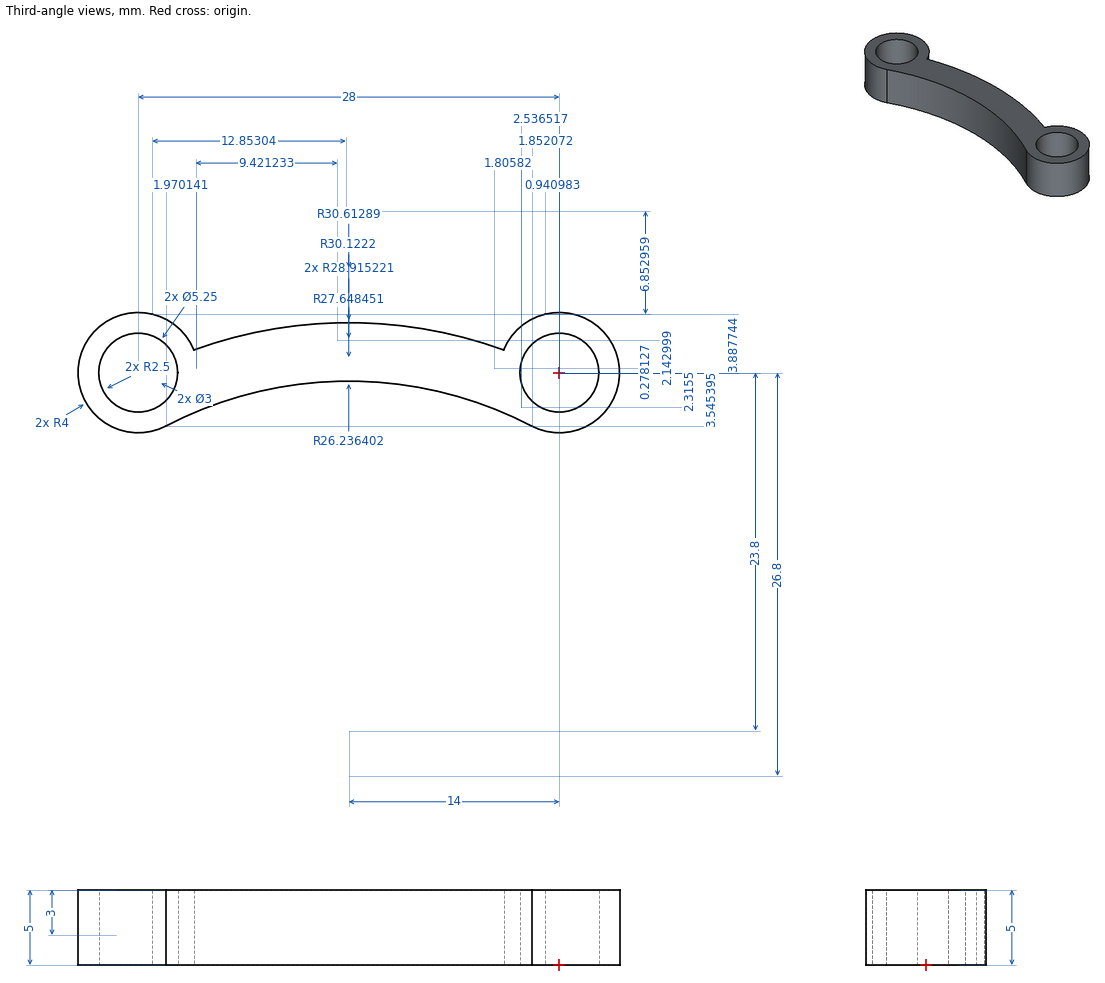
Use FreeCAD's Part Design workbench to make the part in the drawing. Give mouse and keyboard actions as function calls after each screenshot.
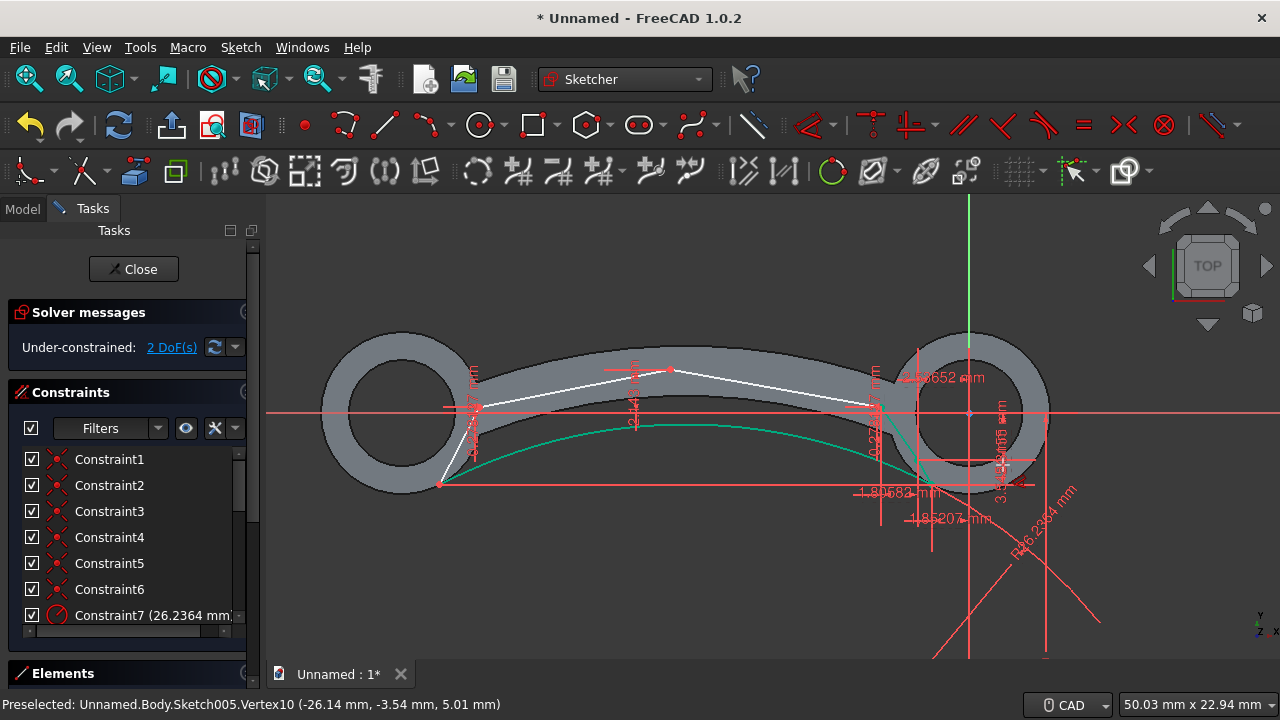
click(613, 381)
click(575, 336)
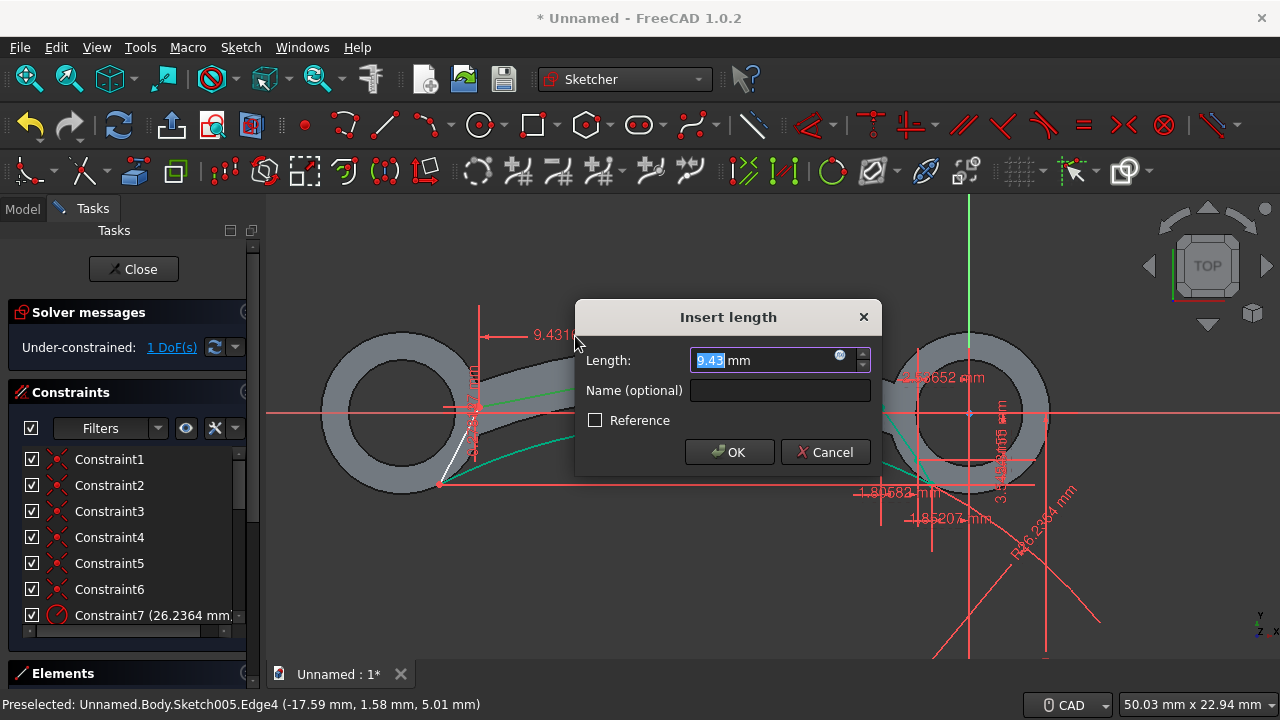
text(9.421233)
key(Return)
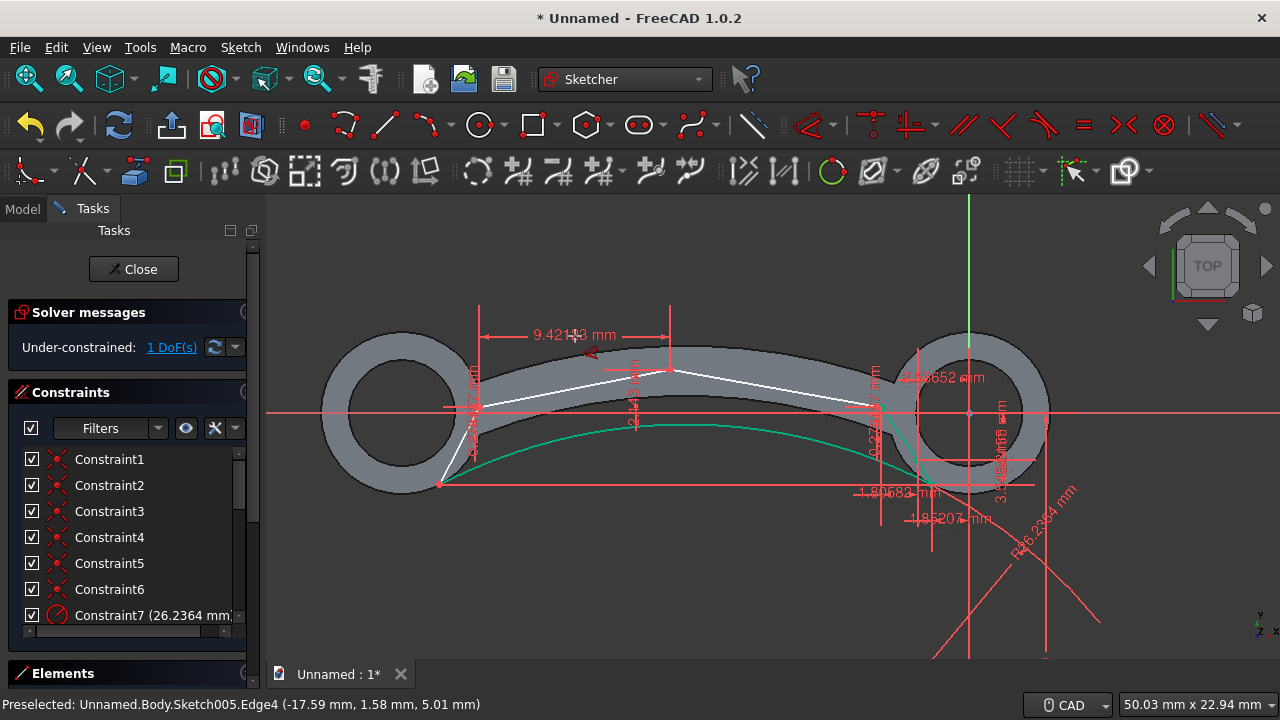
click(467, 431)
click(459, 519)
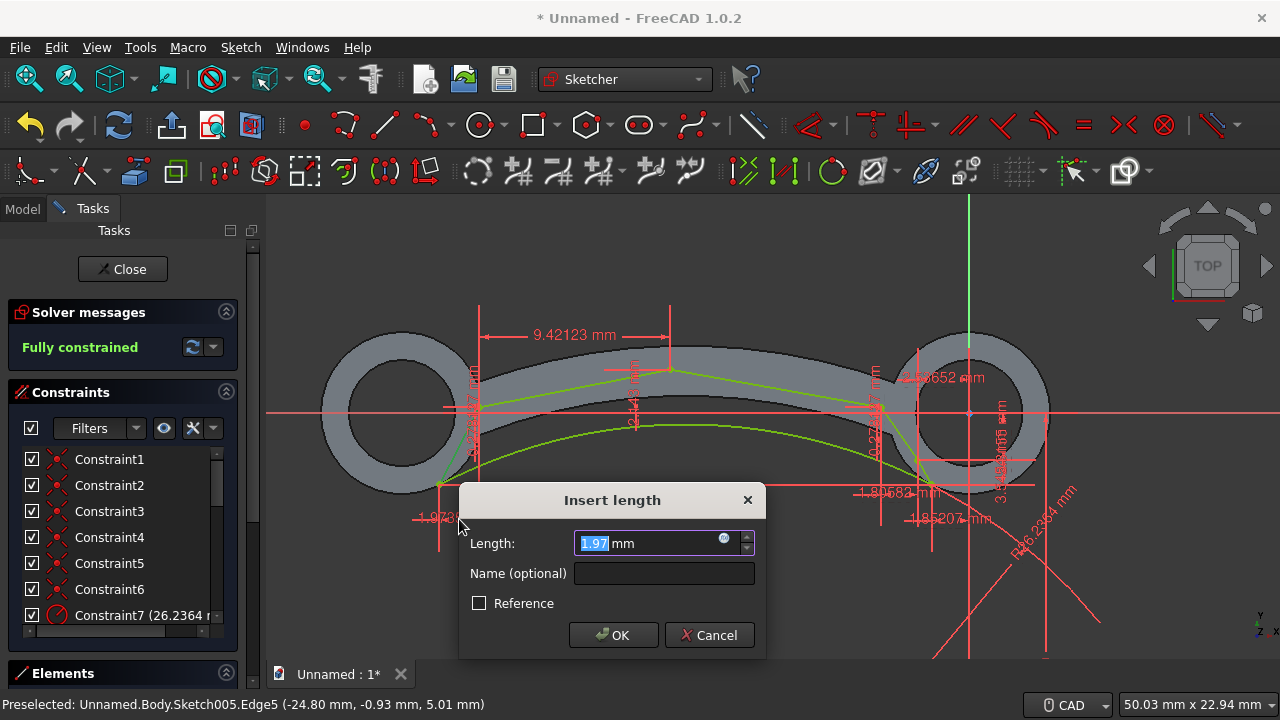
text(1.970141)
key(Return)
key(Escape)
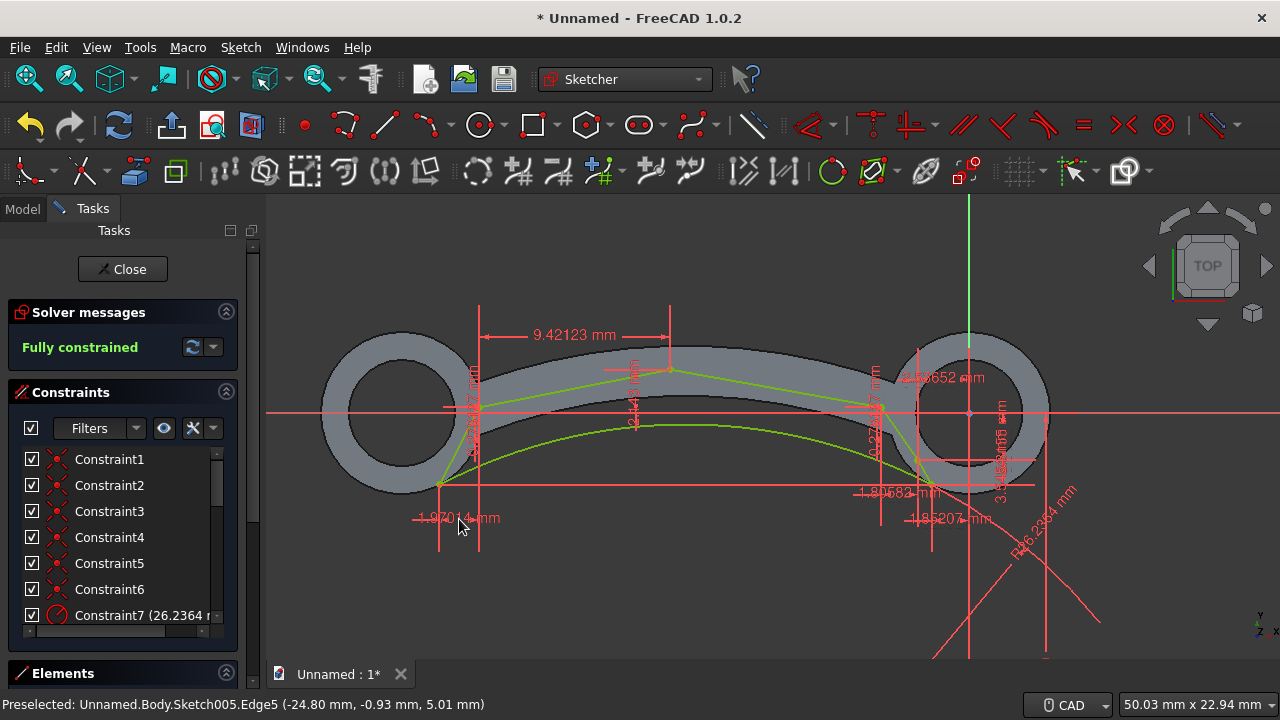
click(123, 269)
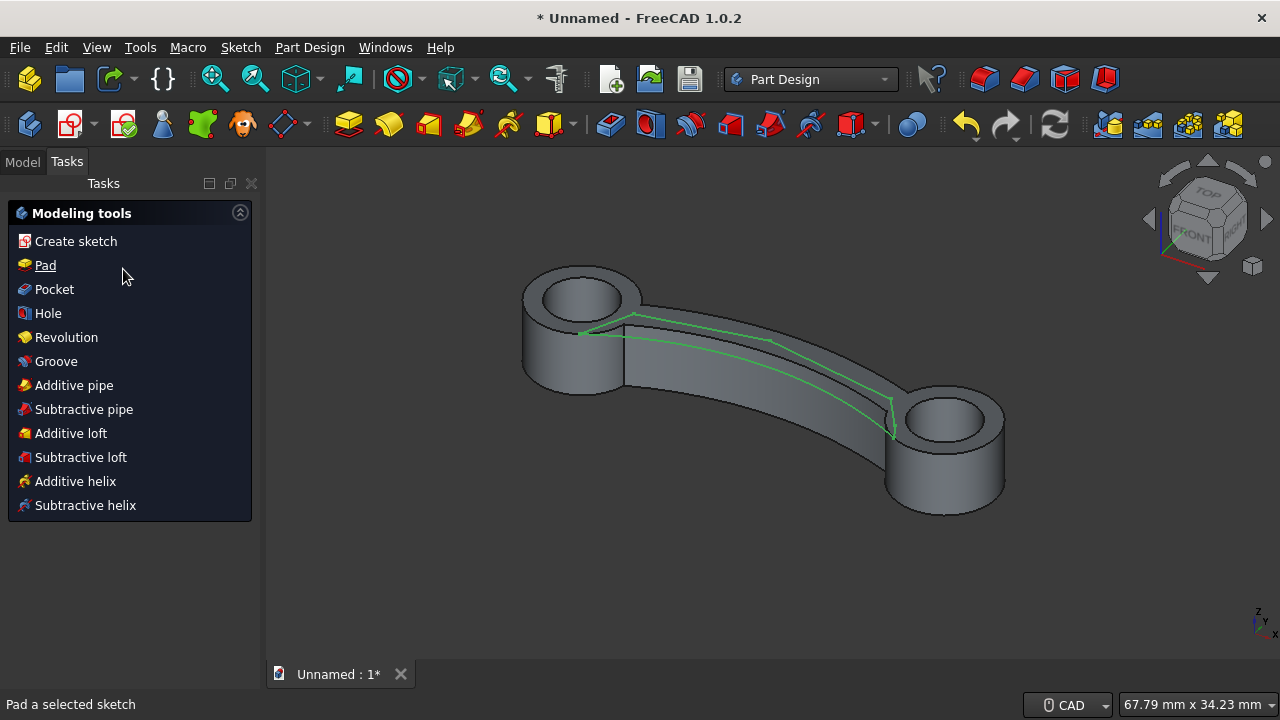
click(350, 124)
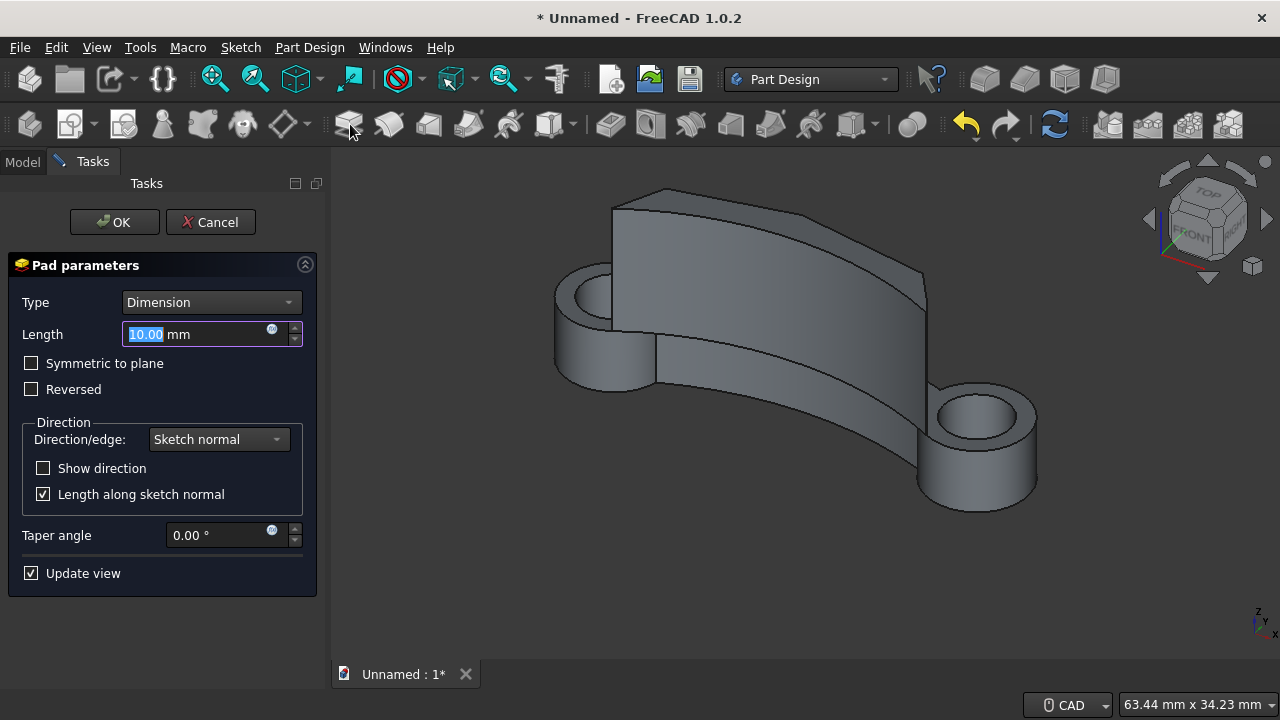
text(5)
key(Tab)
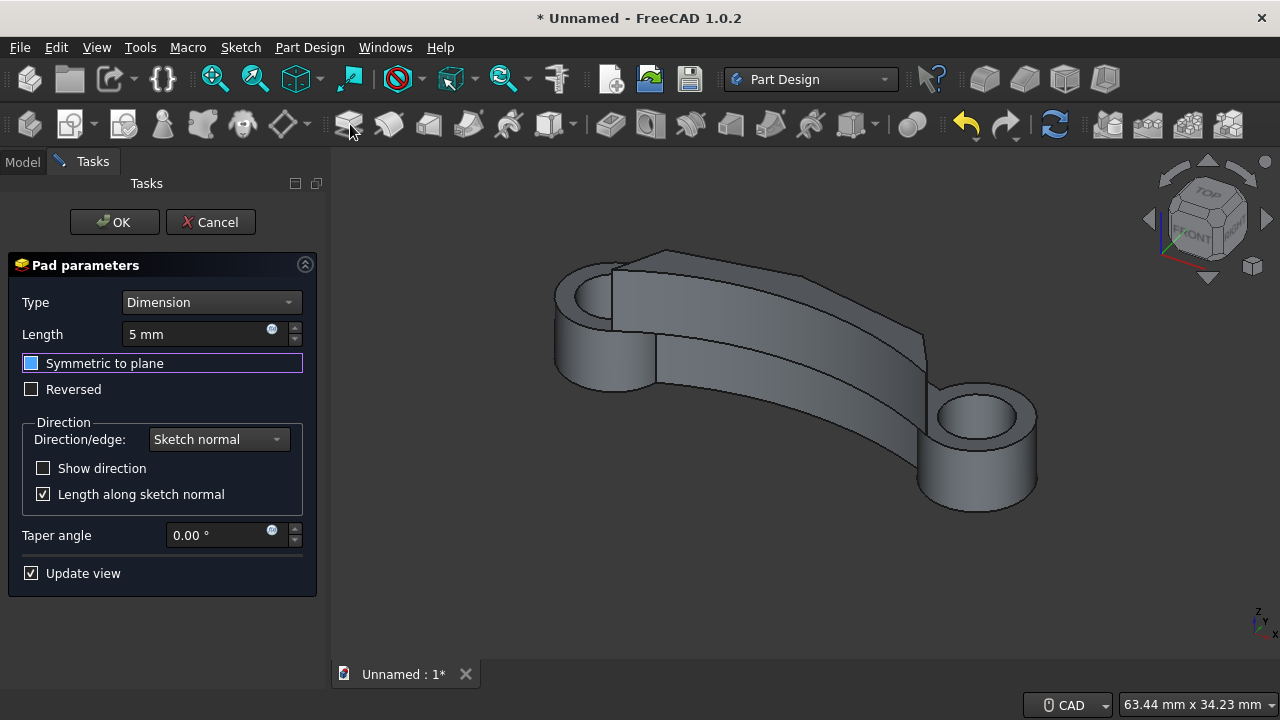
click(30, 389)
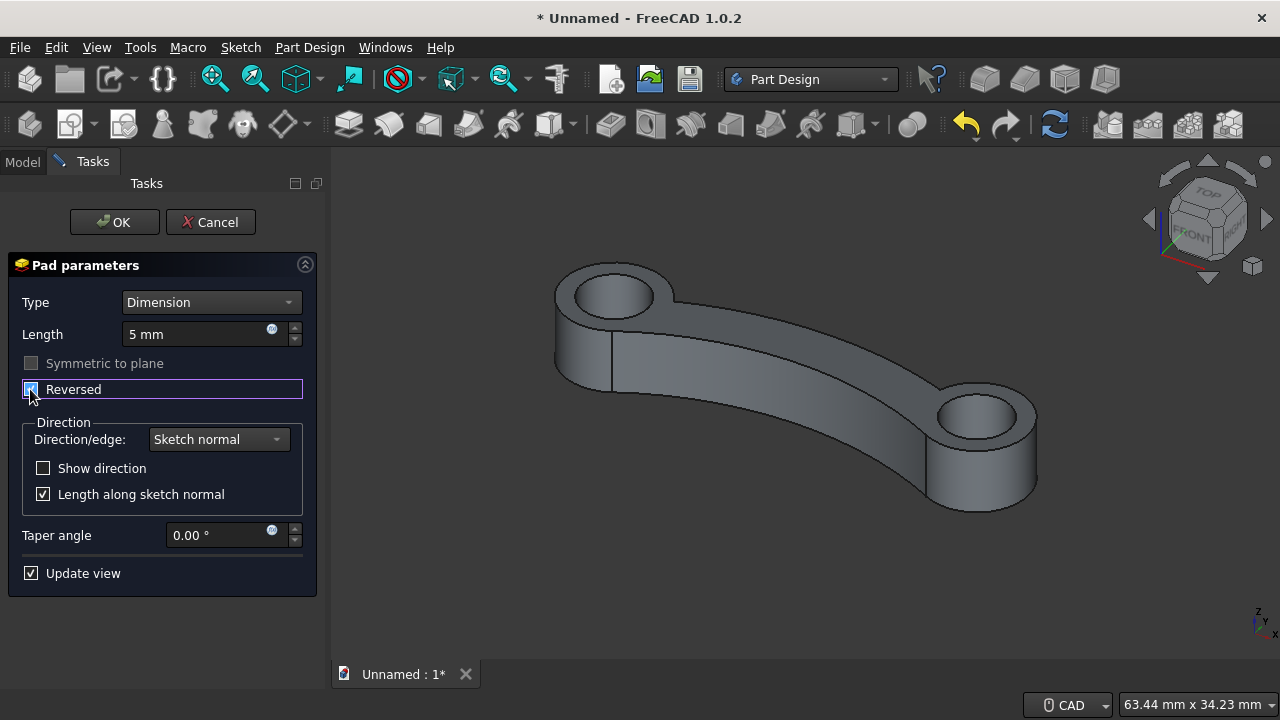
click(115, 222)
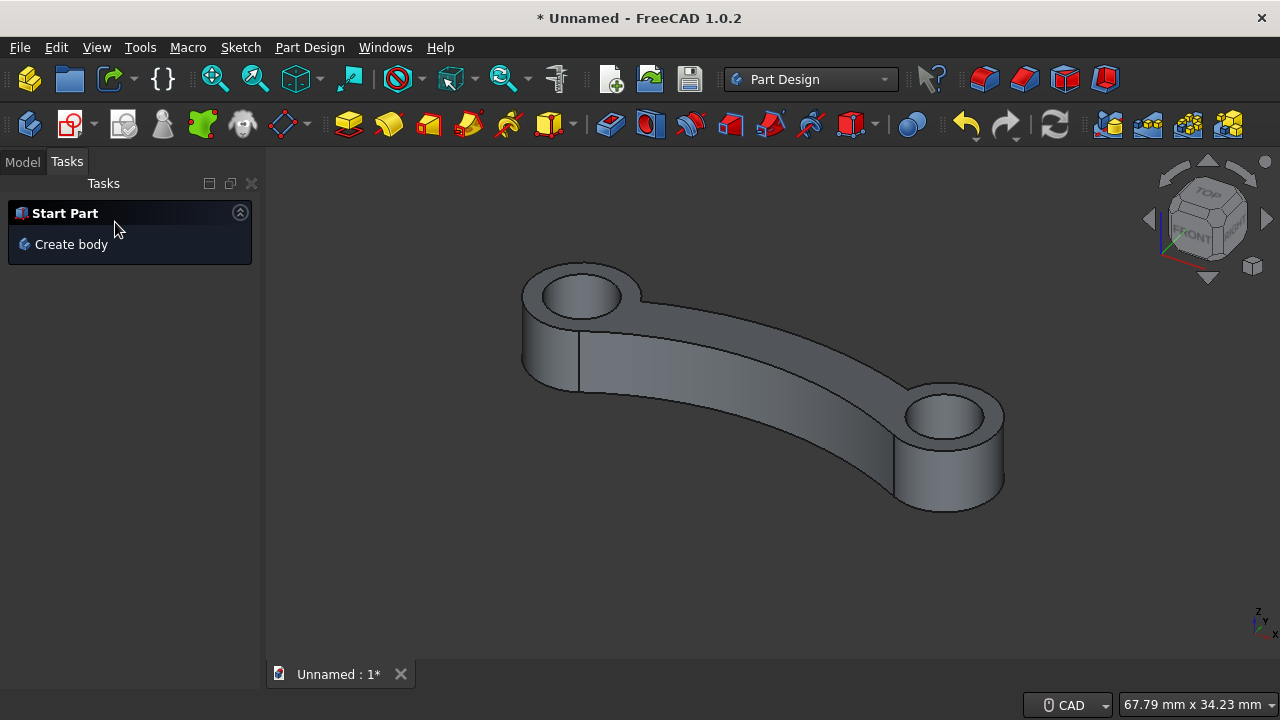
key(0)